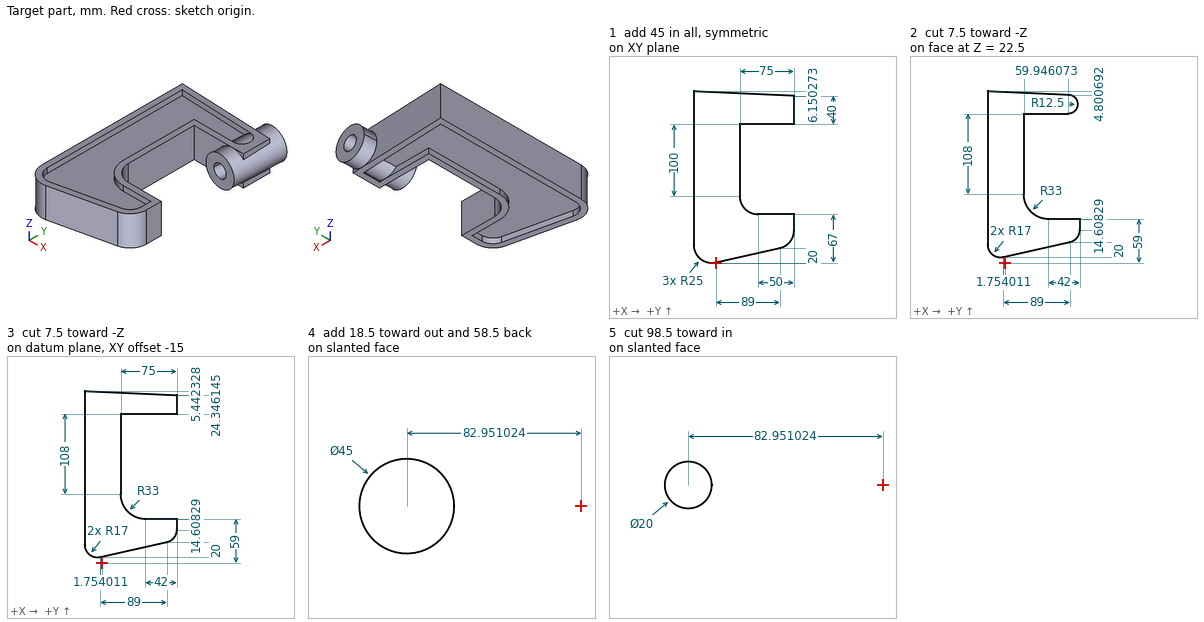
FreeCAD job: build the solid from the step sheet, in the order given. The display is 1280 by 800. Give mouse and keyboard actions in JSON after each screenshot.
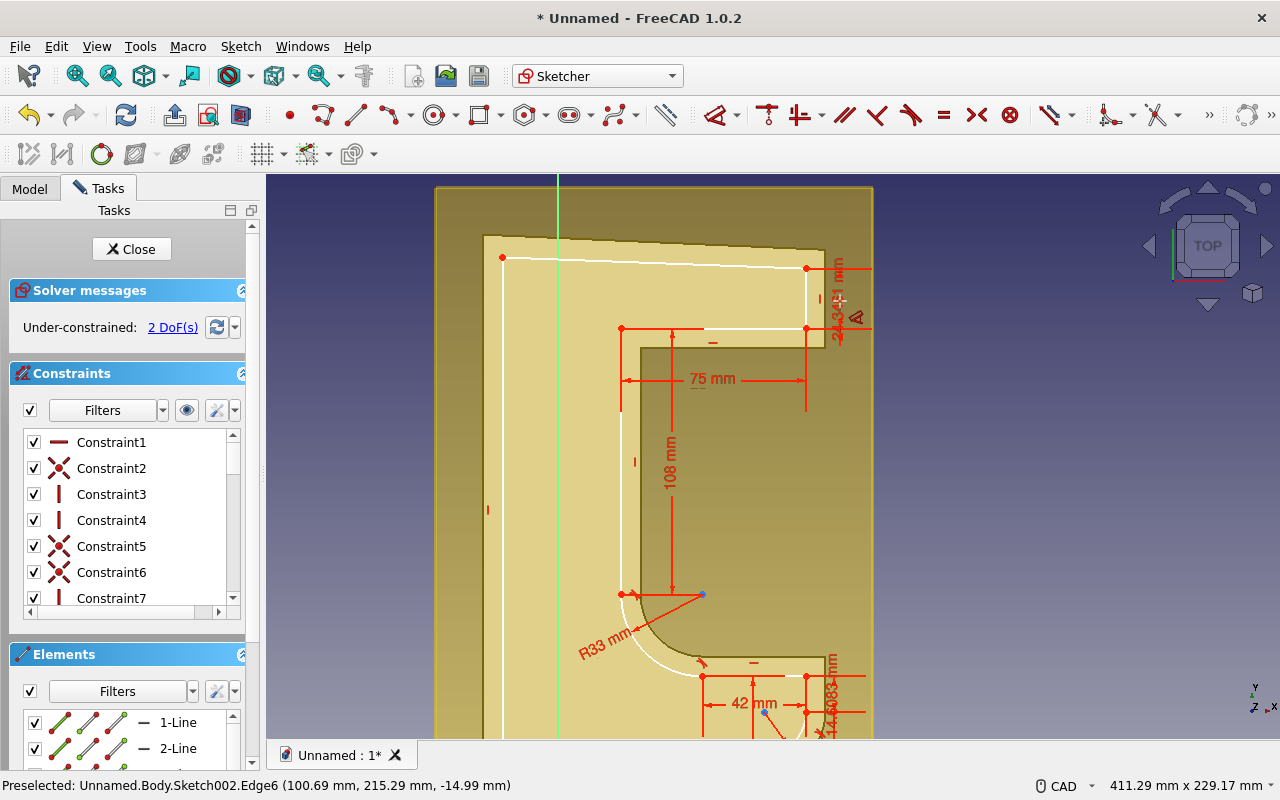
{"action": "scroll", "coordinate": [807, 290], "scroll_direction": "down", "scroll_amount": 2}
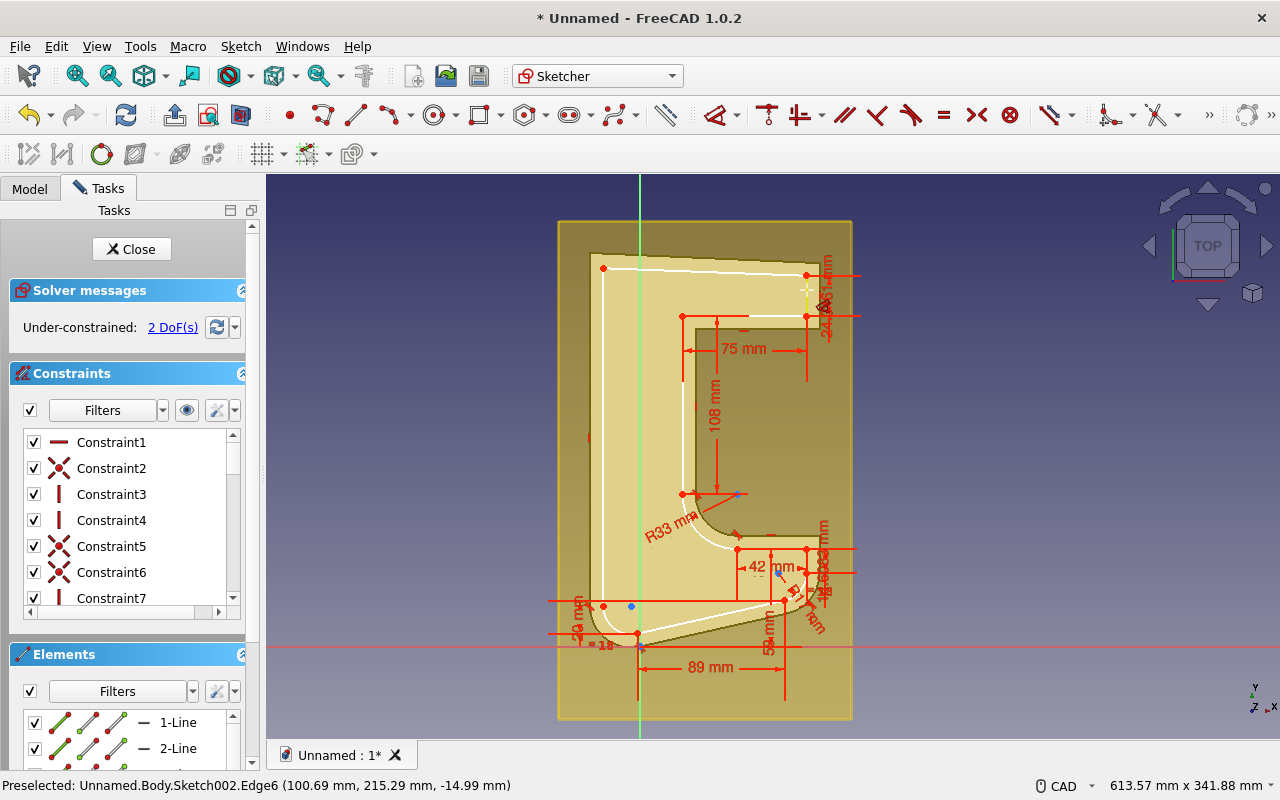
{"action": "scroll", "coordinate": [638, 634], "scroll_direction": "up", "scroll_amount": 14}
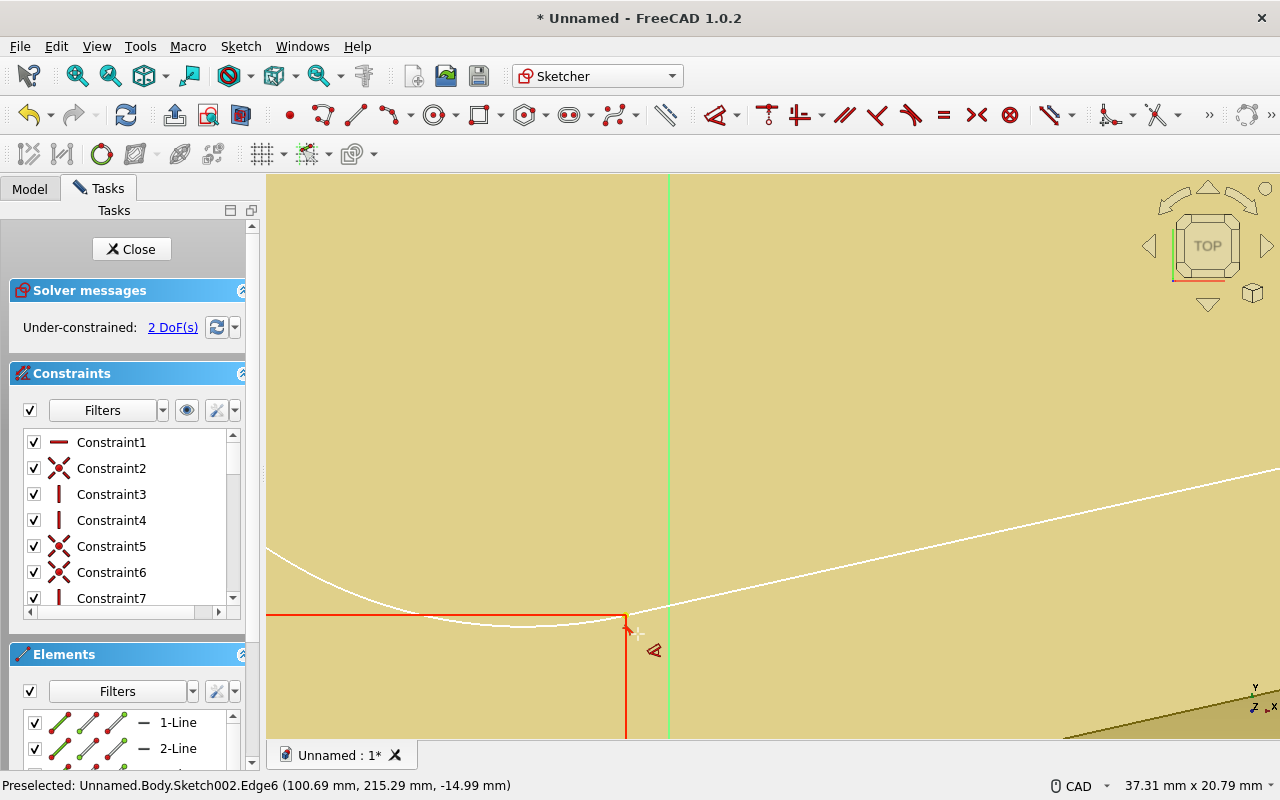
{"action": "left_click", "coordinate": [626, 615]}
{"action": "left_click", "coordinate": [647, 581]}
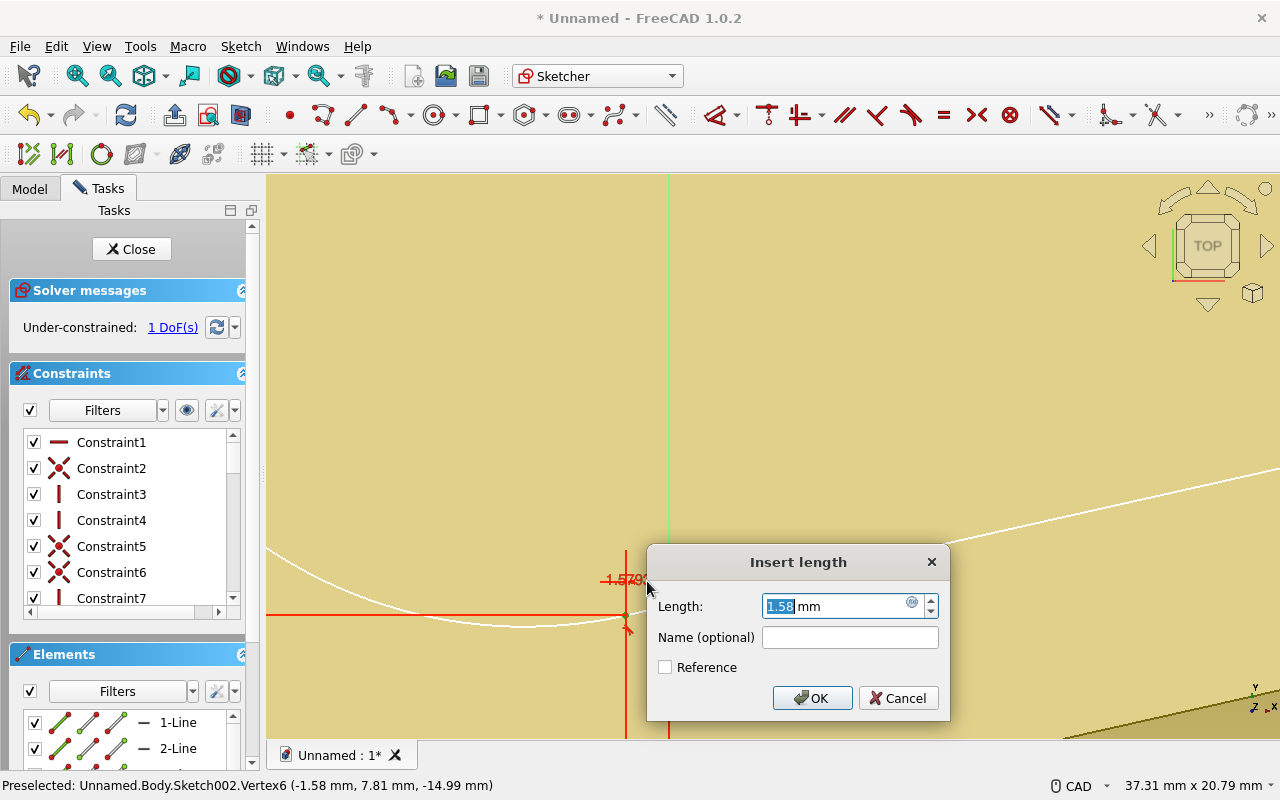
{"action": "type", "text": "1.754011"}
{"action": "key", "text": "Return"}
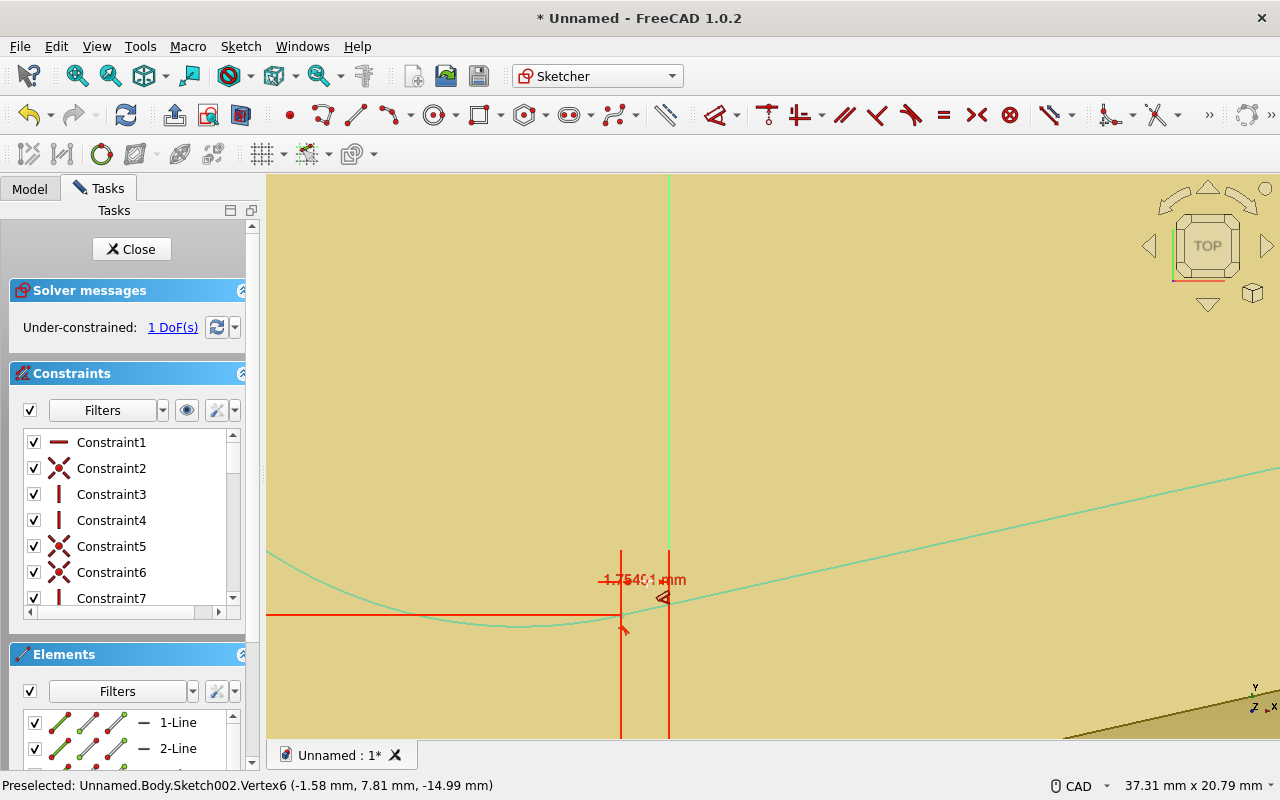
{"action": "scroll", "coordinate": [638, 635], "scroll_direction": "down", "scroll_amount": 14}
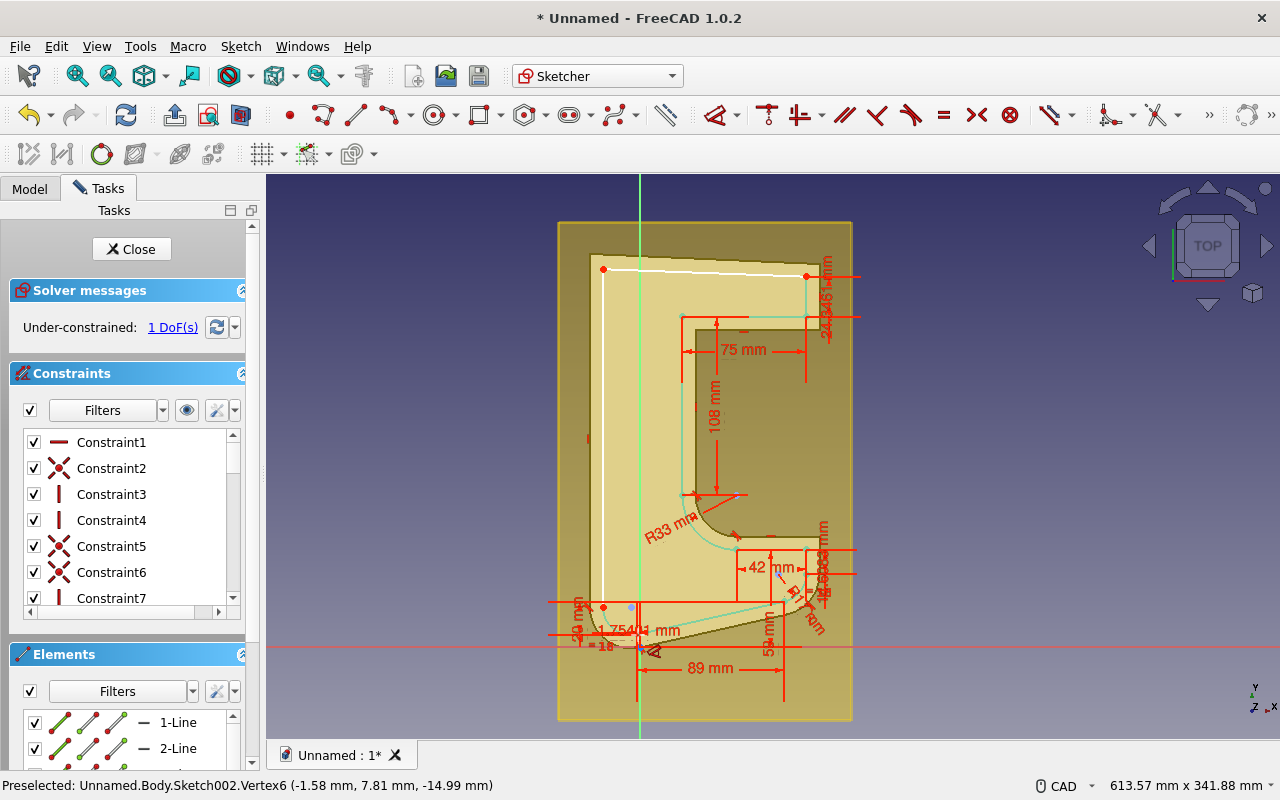
{"action": "scroll", "coordinate": [664, 271], "scroll_direction": "up", "scroll_amount": 8}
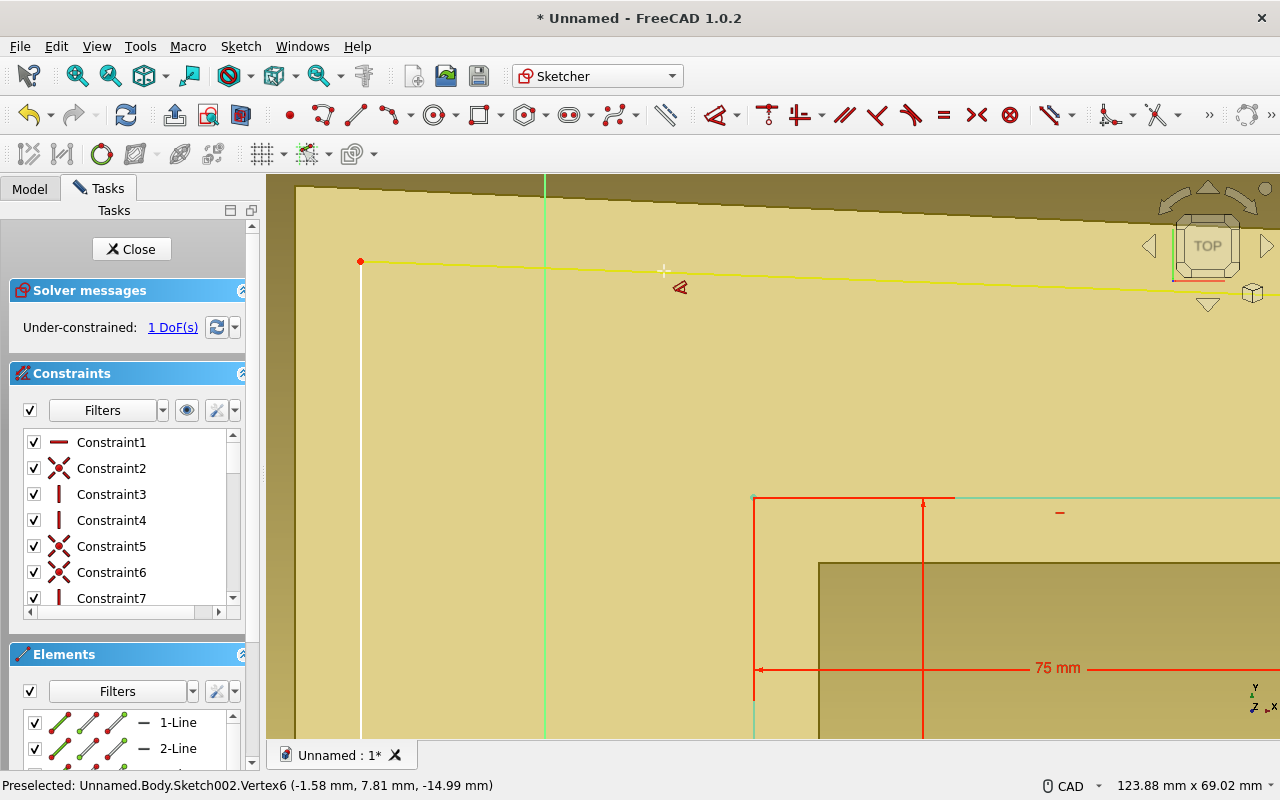
{"action": "left_click", "coordinate": [663, 273]}
{"action": "left_click", "coordinate": [327, 280]}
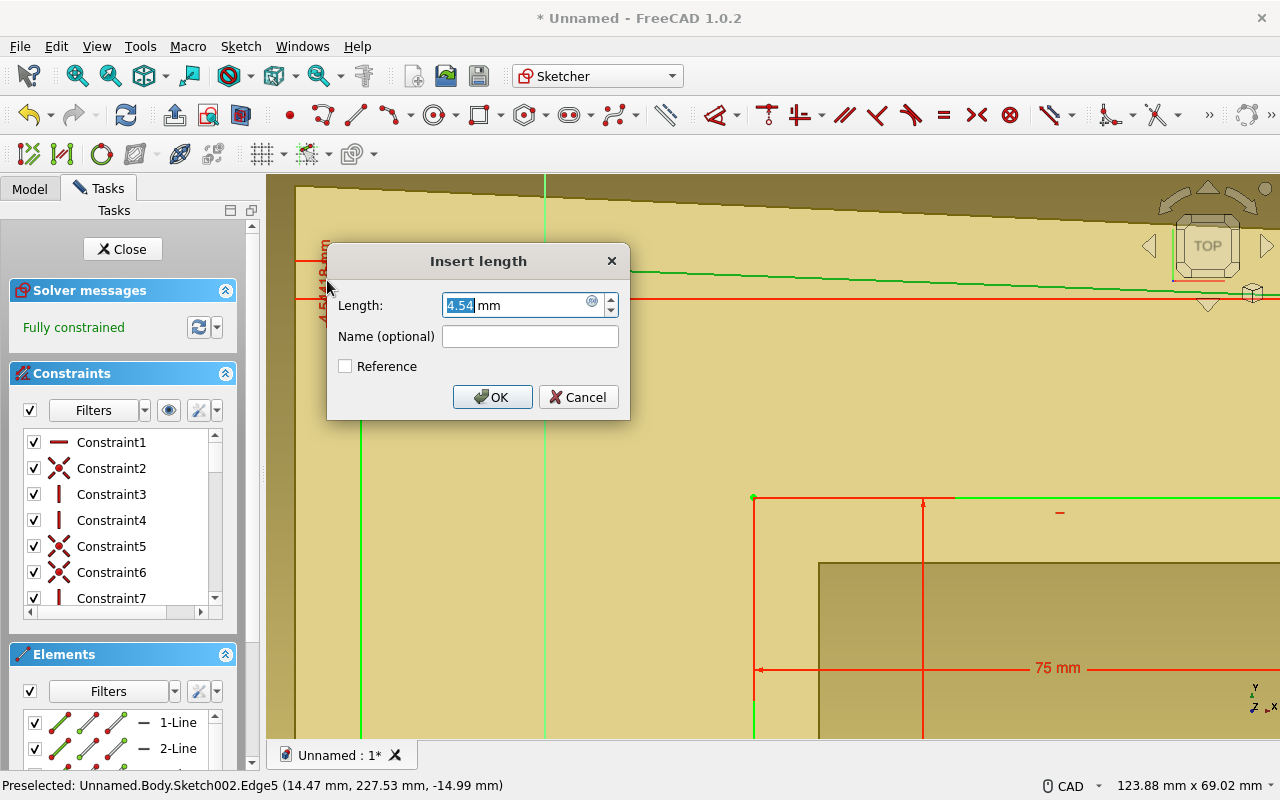
{"action": "type", "text": "5.442328"}
{"action": "key", "text": "Return"}
{"action": "key", "text": "Escape"}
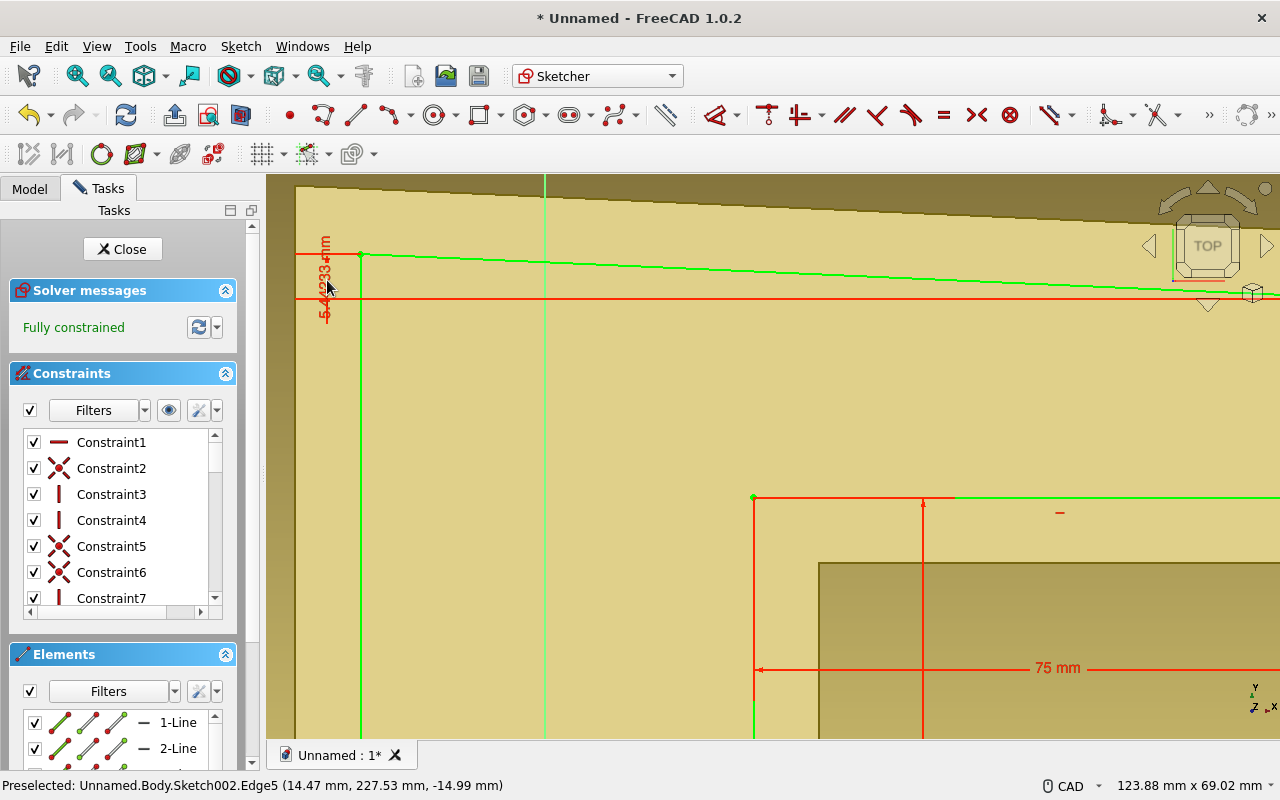
{"action": "left_click", "coordinate": [123, 249]}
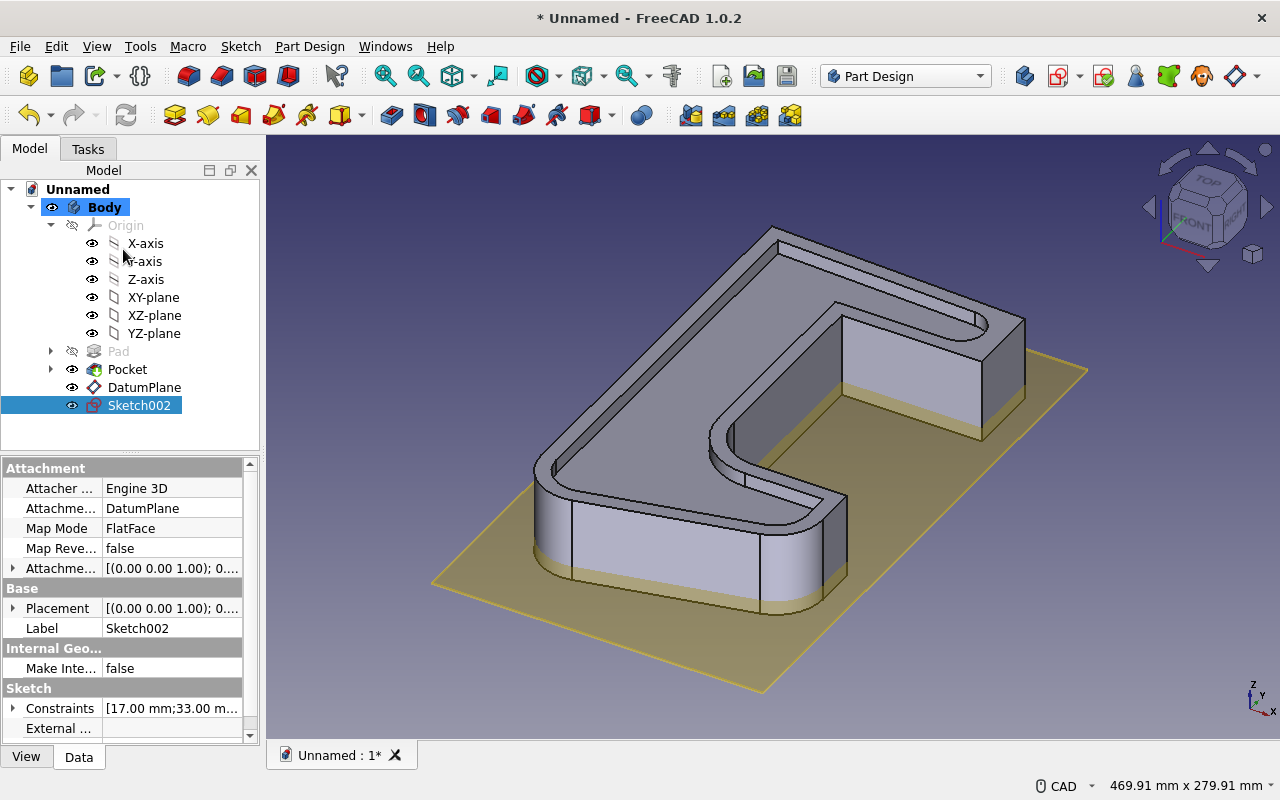
{"action": "left_click", "coordinate": [392, 116]}